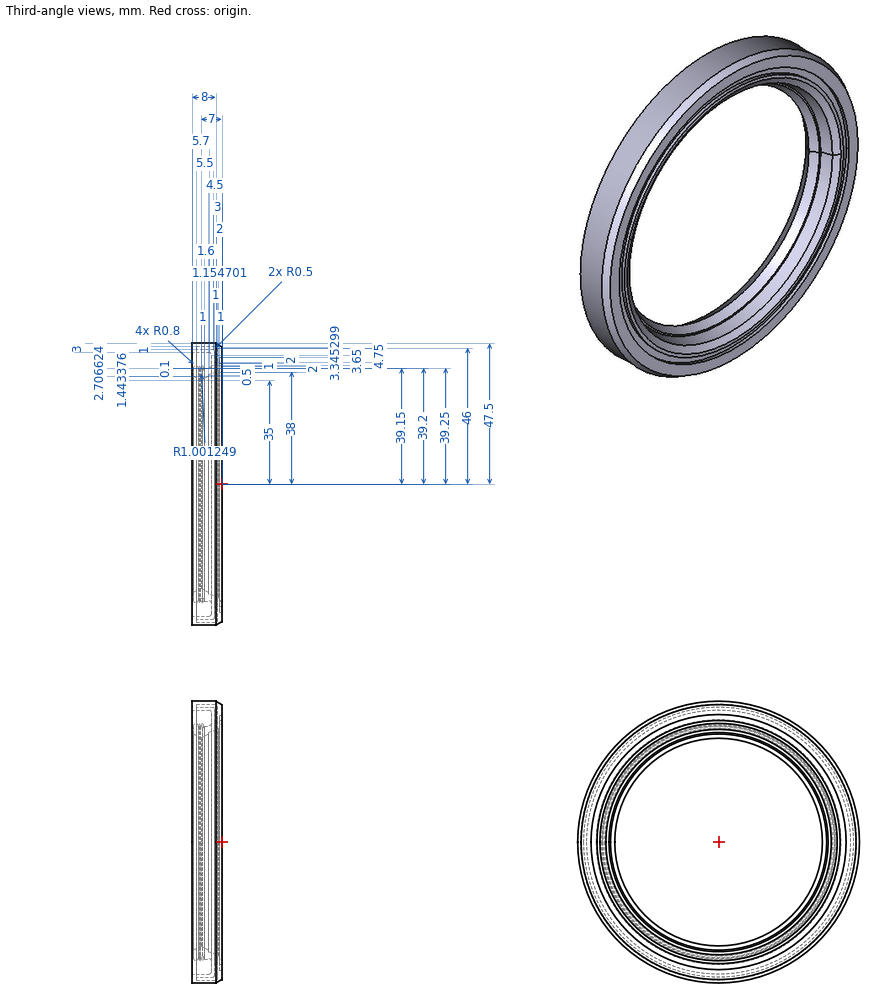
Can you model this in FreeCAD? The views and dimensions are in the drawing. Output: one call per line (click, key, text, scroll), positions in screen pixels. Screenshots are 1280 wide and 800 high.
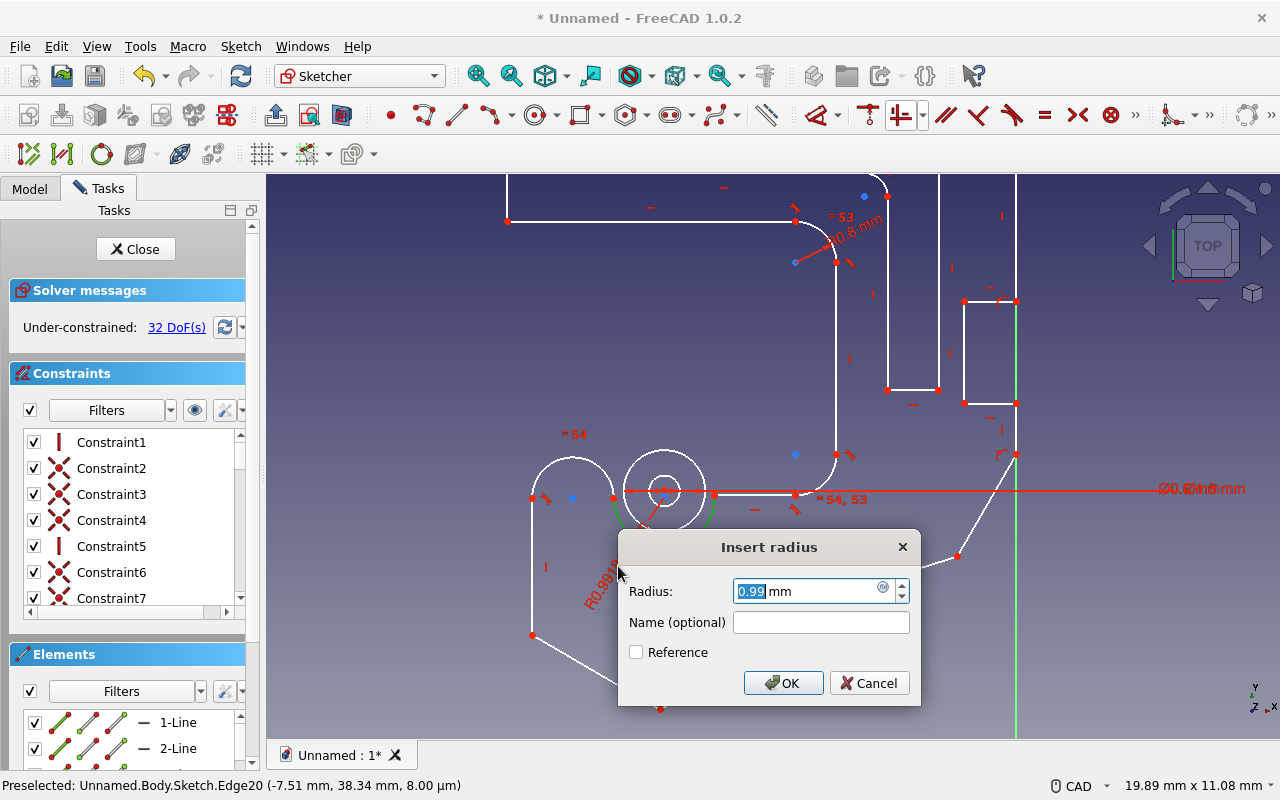
text(1.001249)
key(Return)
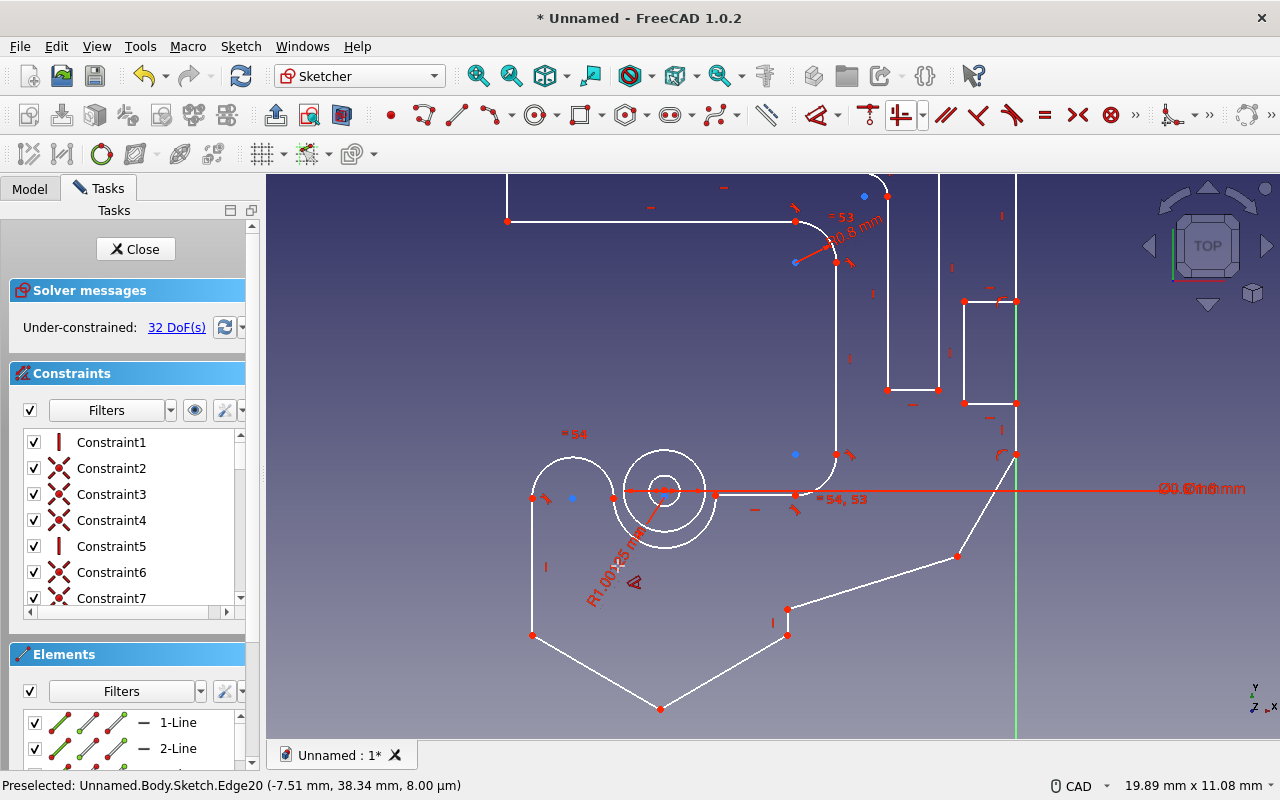
scroll(635, 539, down, 3)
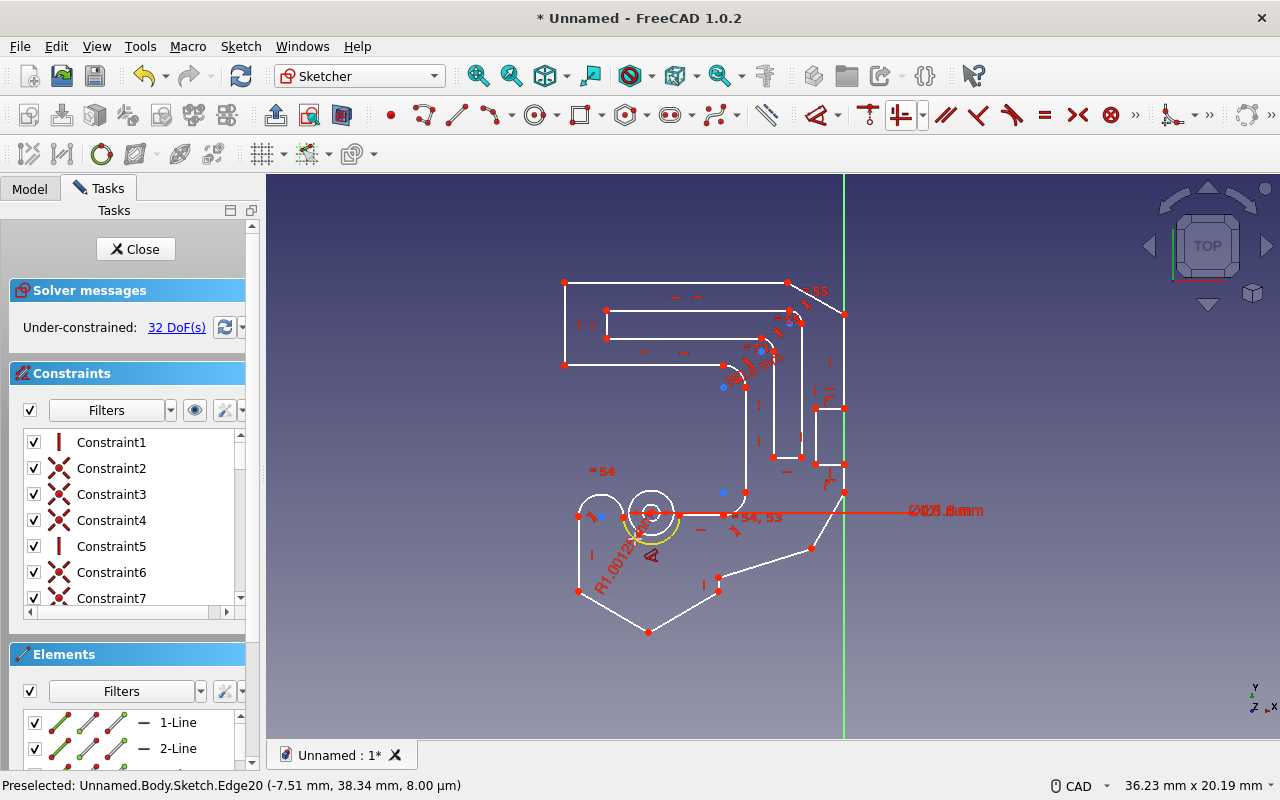
scroll(800, 318, up, 6)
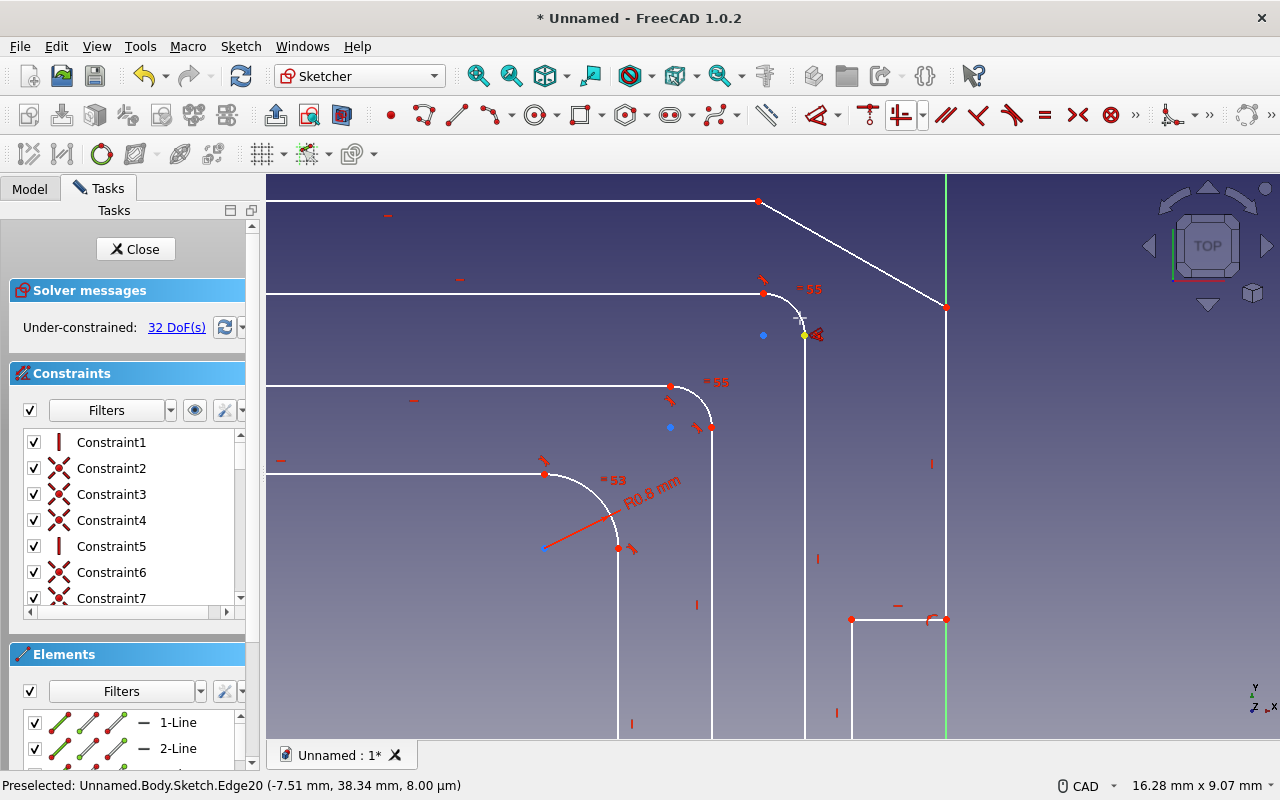
click(800, 316)
click(828, 301)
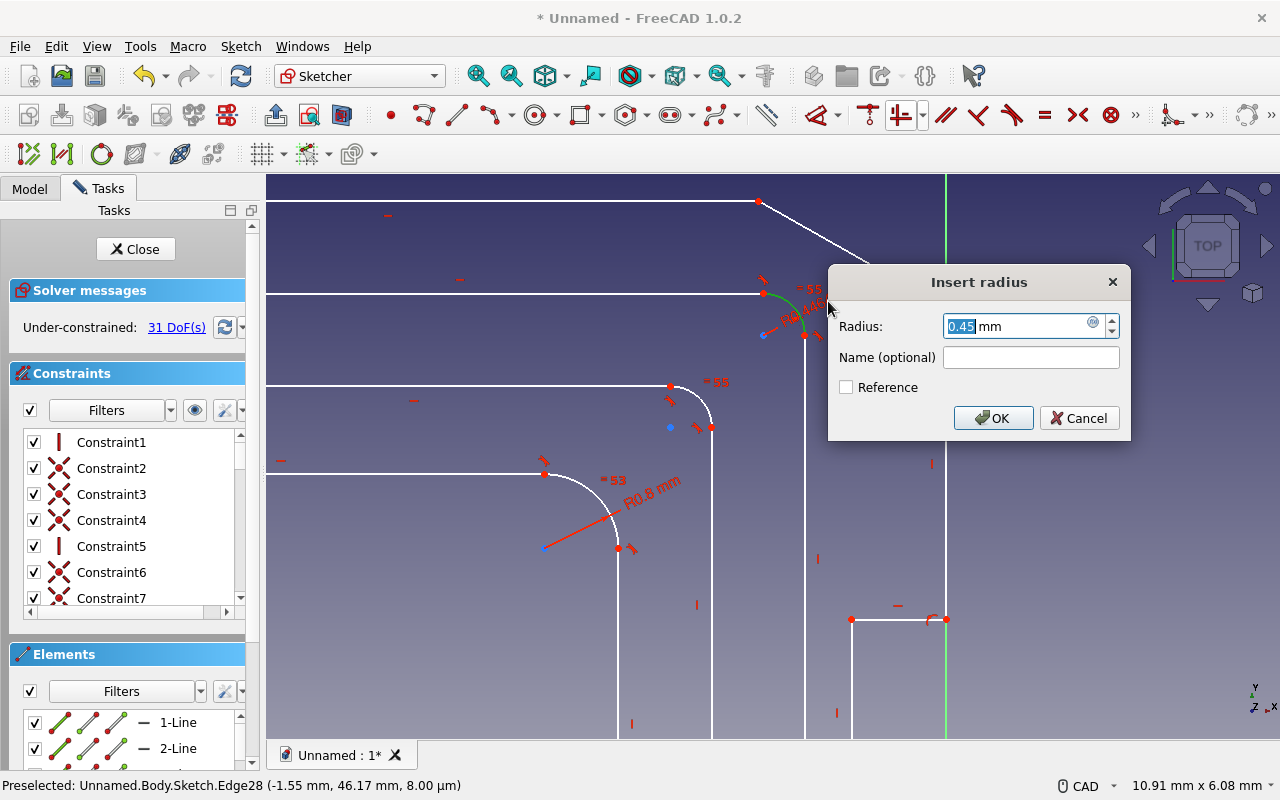
text(0.5)
key(Return)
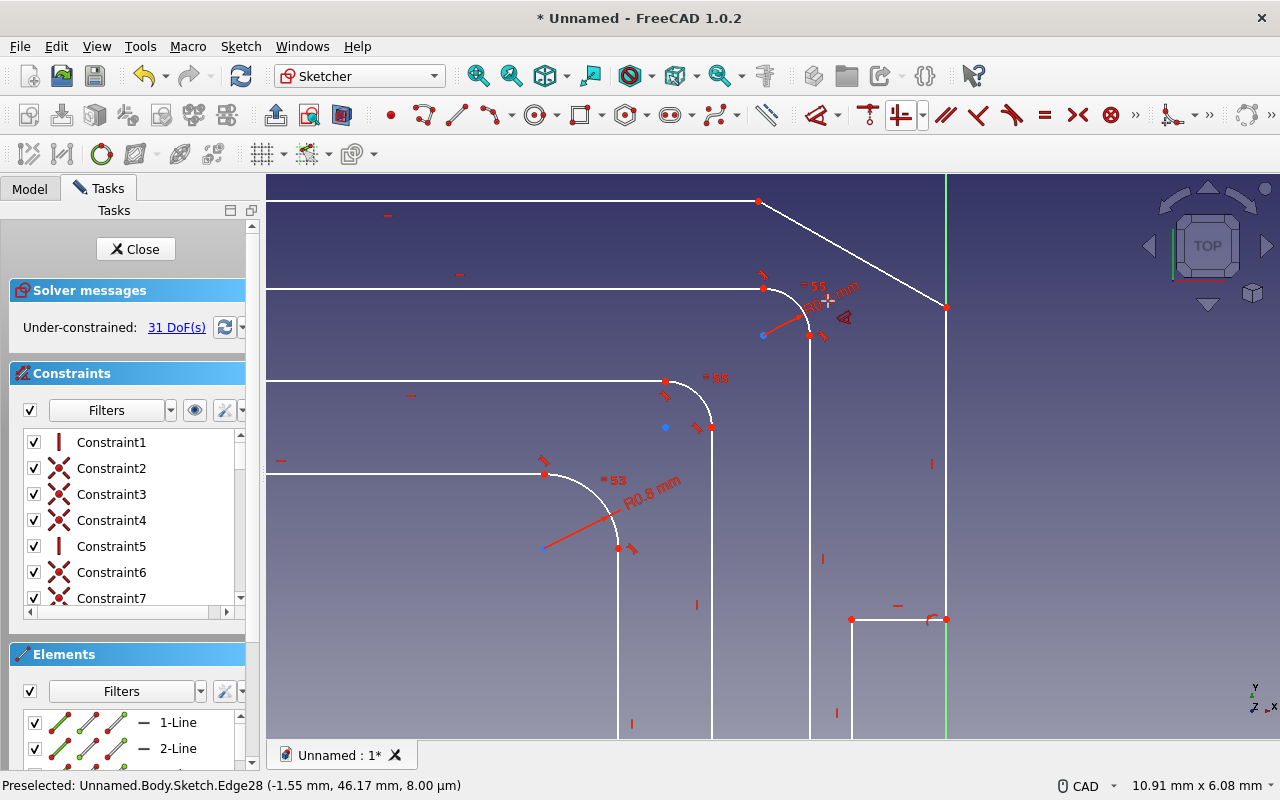
scroll(801, 318, down, 6)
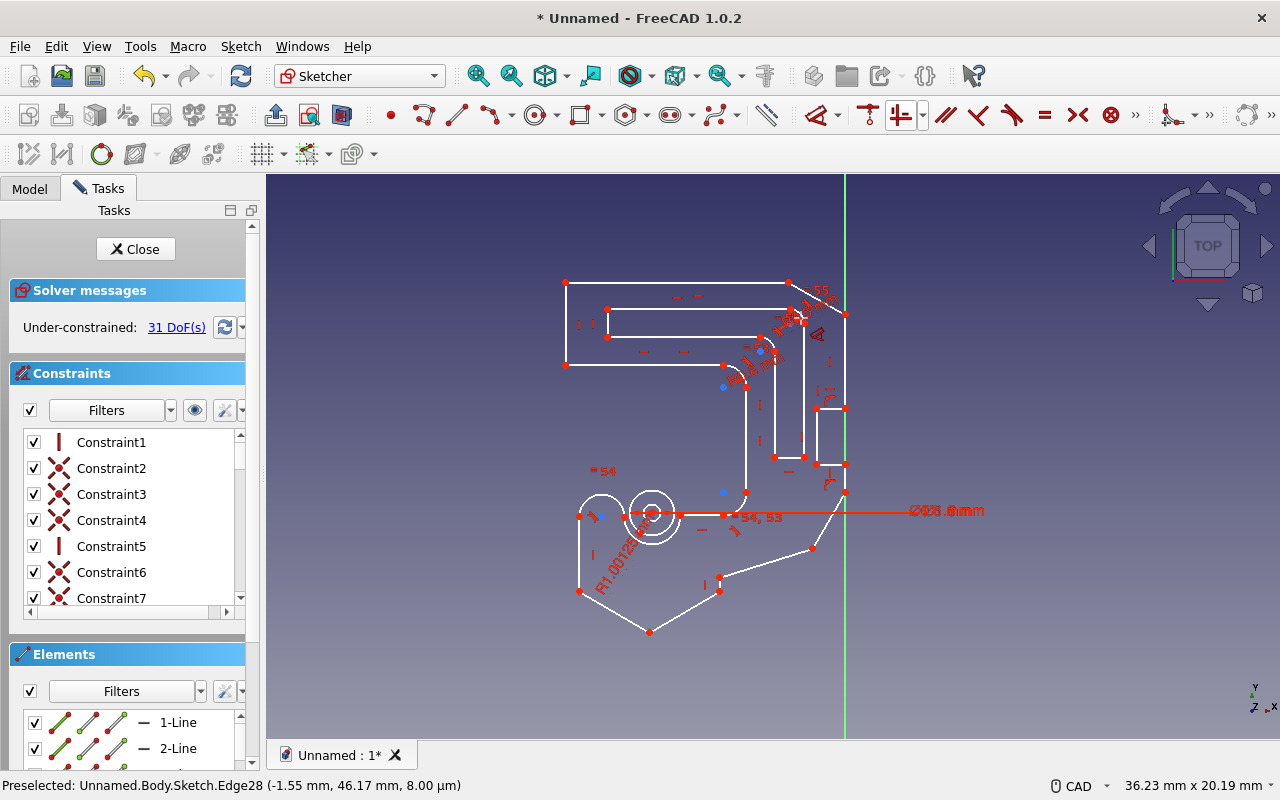
scroll(845, 485, up, 3)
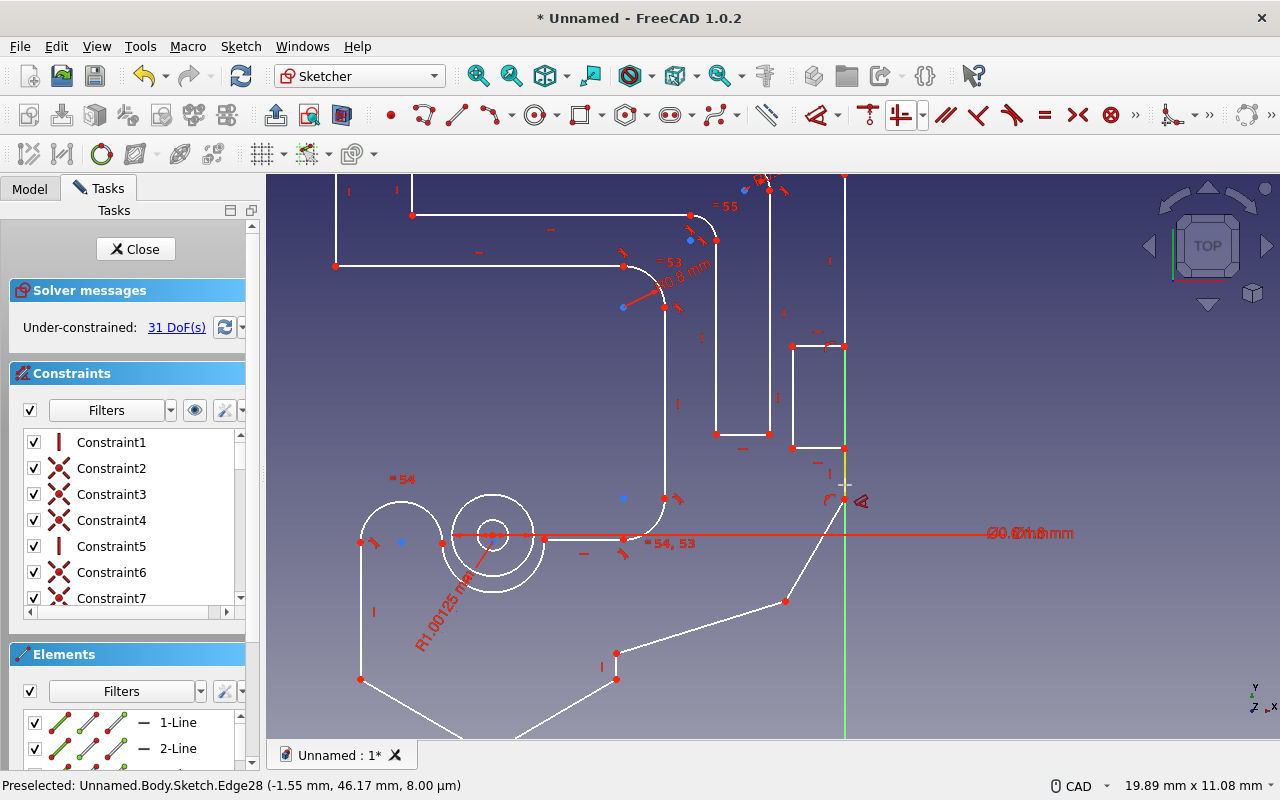
click(845, 484)
click(879, 474)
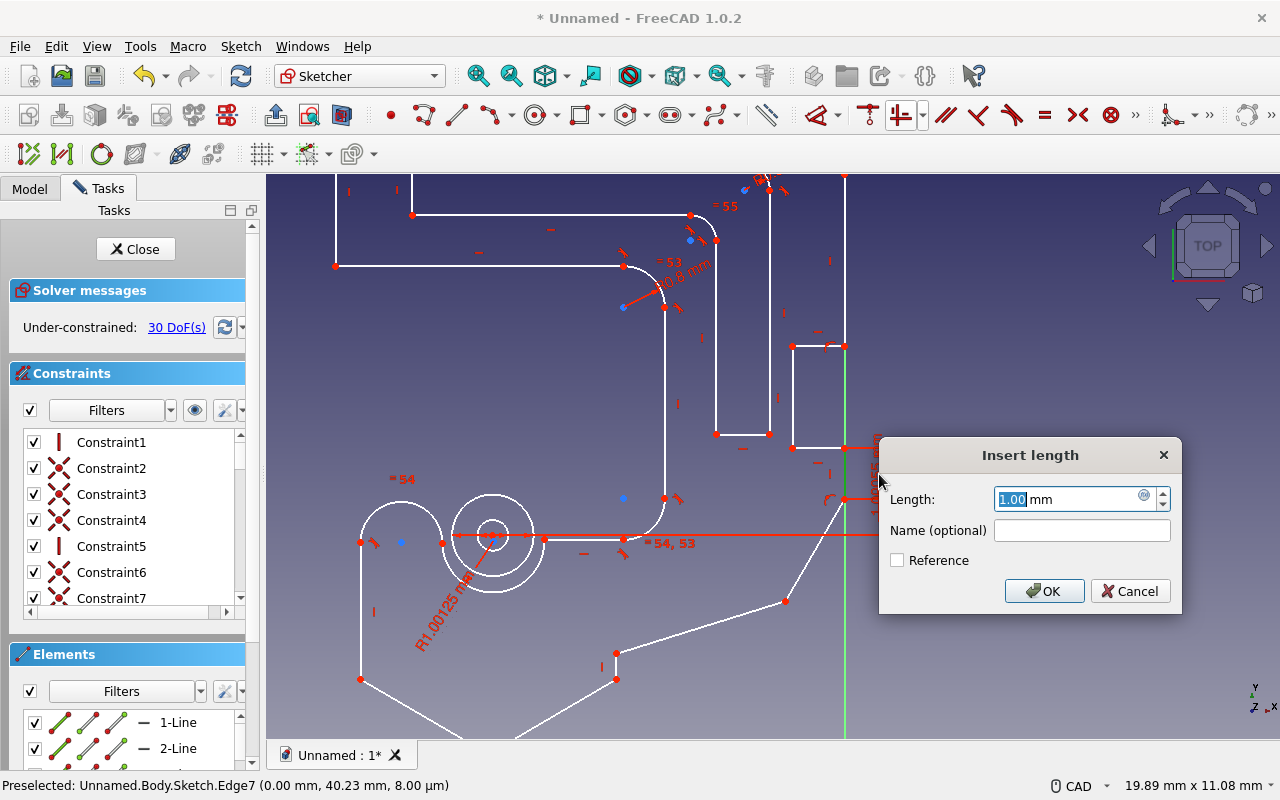
text(1)
key(Return)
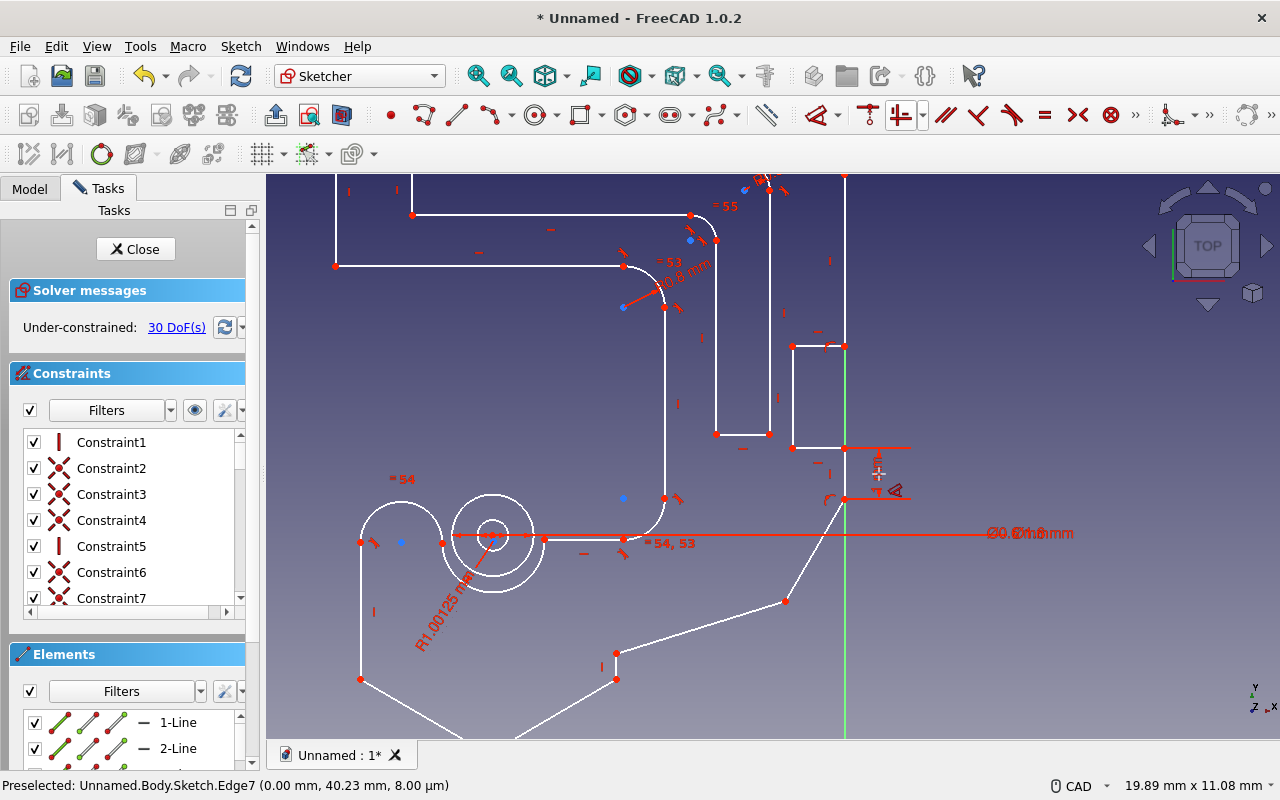
click(829, 448)
click(807, 482)